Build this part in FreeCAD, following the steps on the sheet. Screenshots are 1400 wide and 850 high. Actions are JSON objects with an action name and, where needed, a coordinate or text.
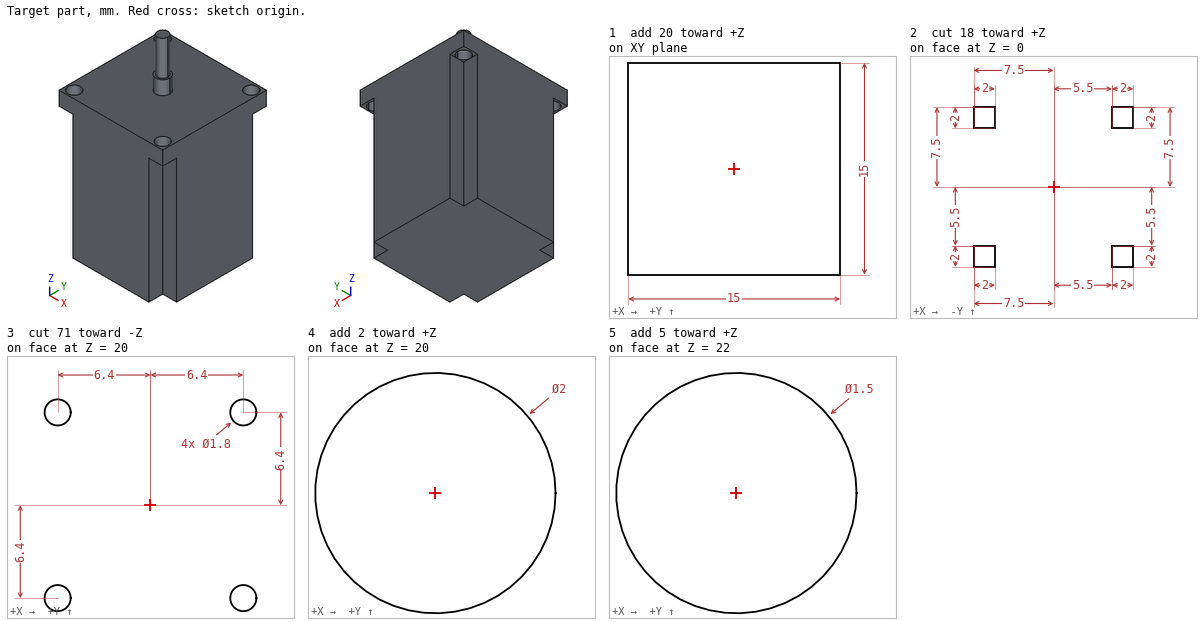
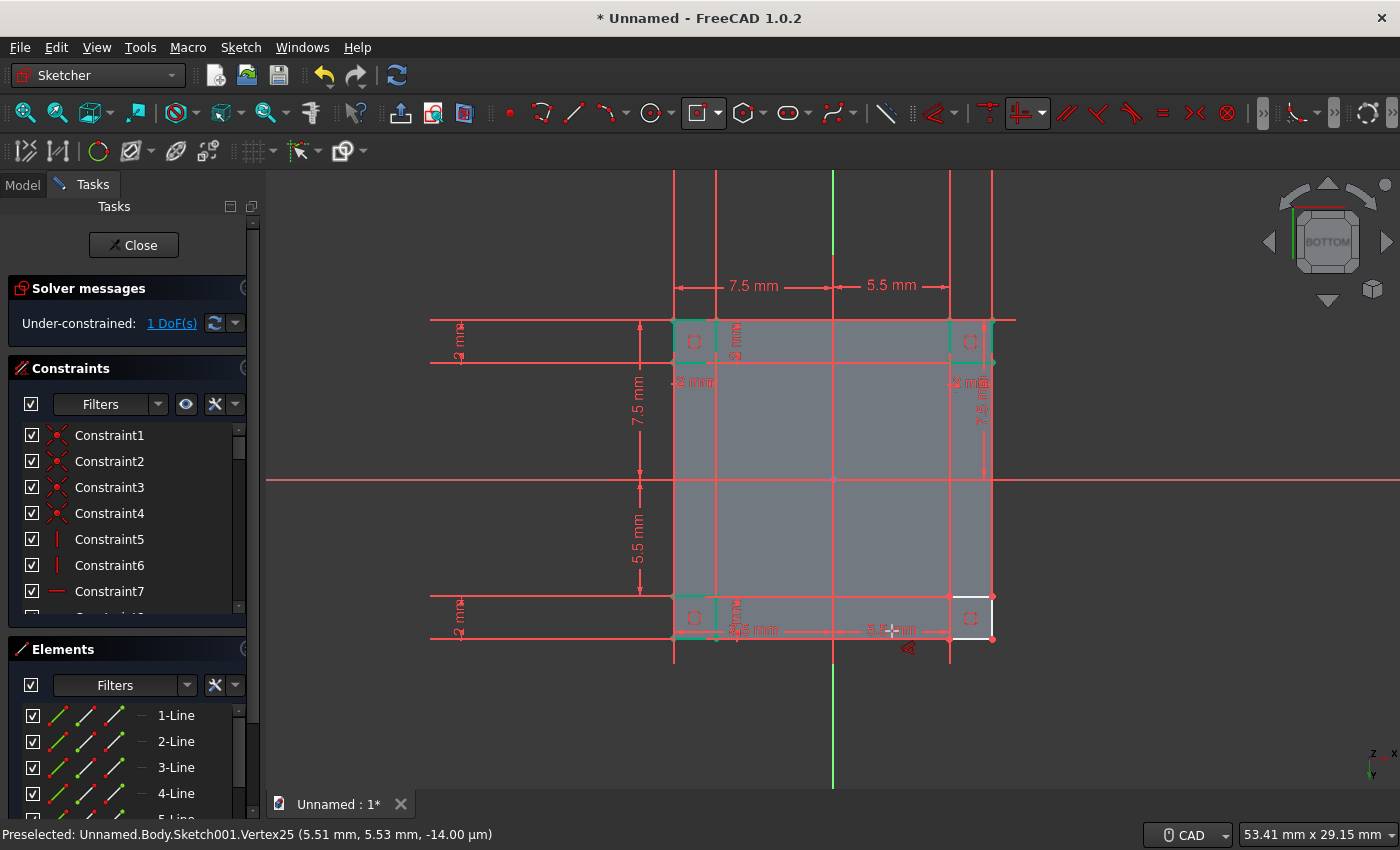
{"action": "left_click", "coordinate": [950, 597]}
{"action": "left_click", "coordinate": [984, 538]}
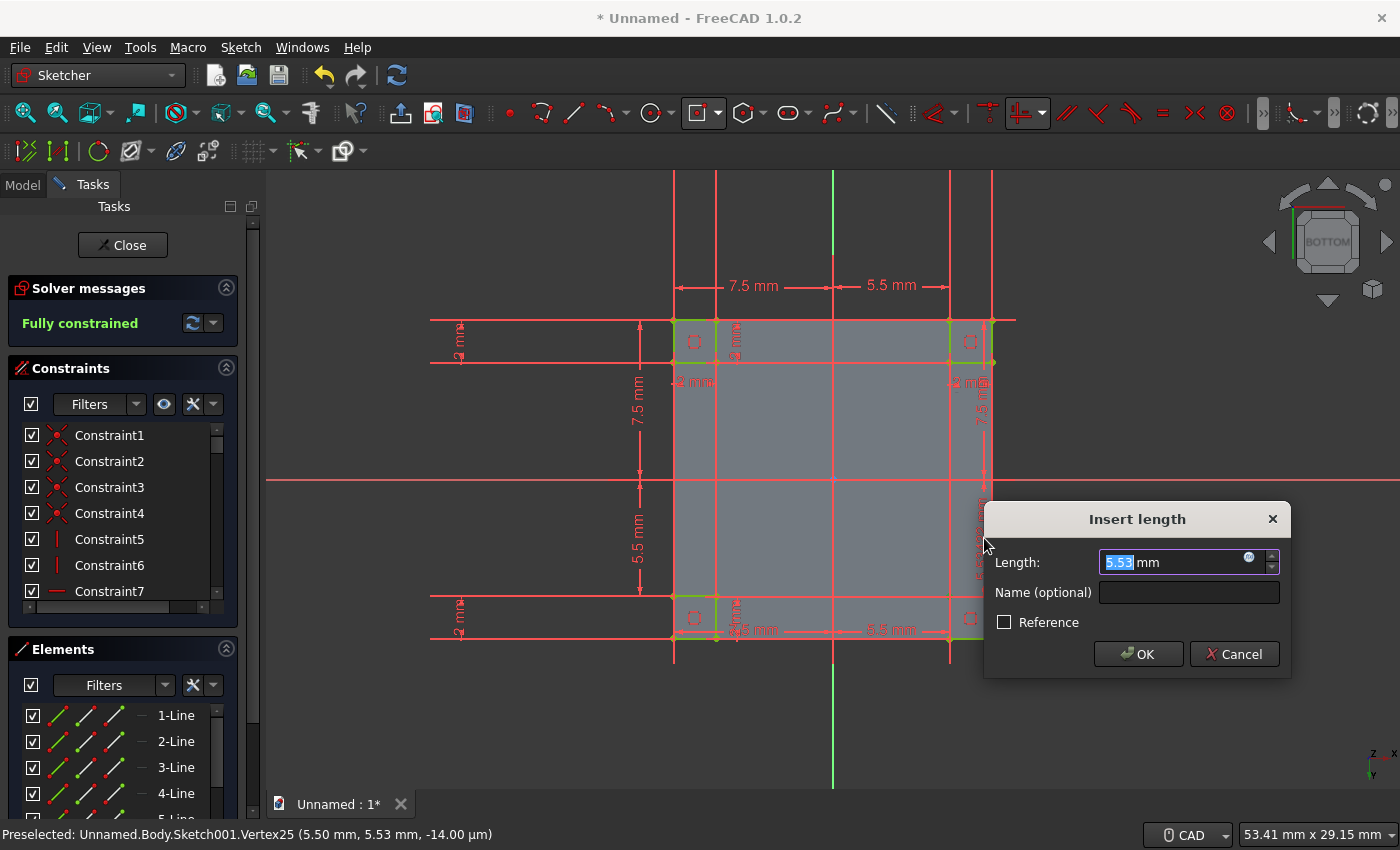
{"action": "type", "text": "5.5"}
{"action": "key", "text": "Return"}
{"action": "key", "text": "Escape"}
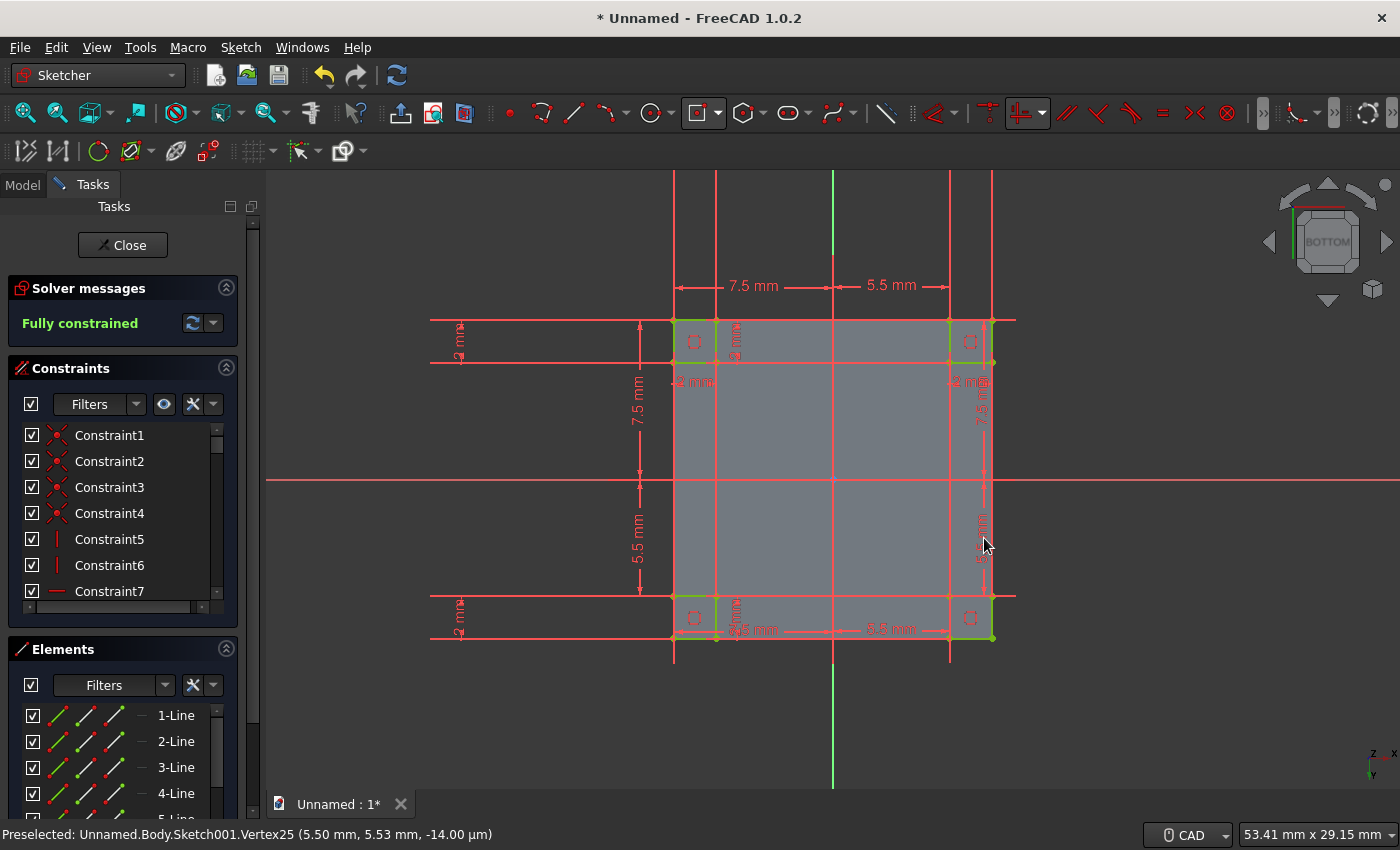
{"action": "left_click", "coordinate": [123, 245]}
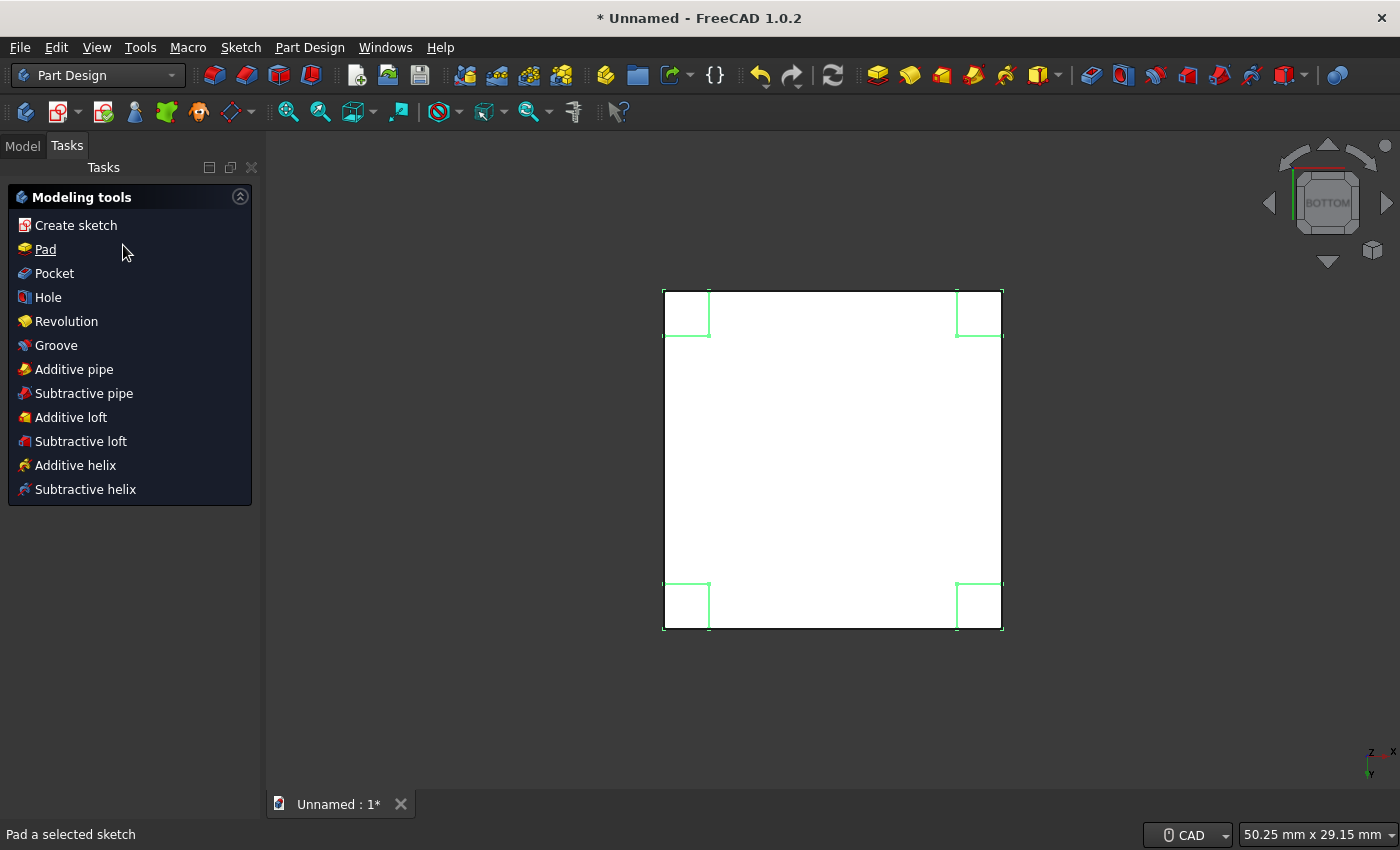
{"action": "left_click", "coordinate": [1092, 76]}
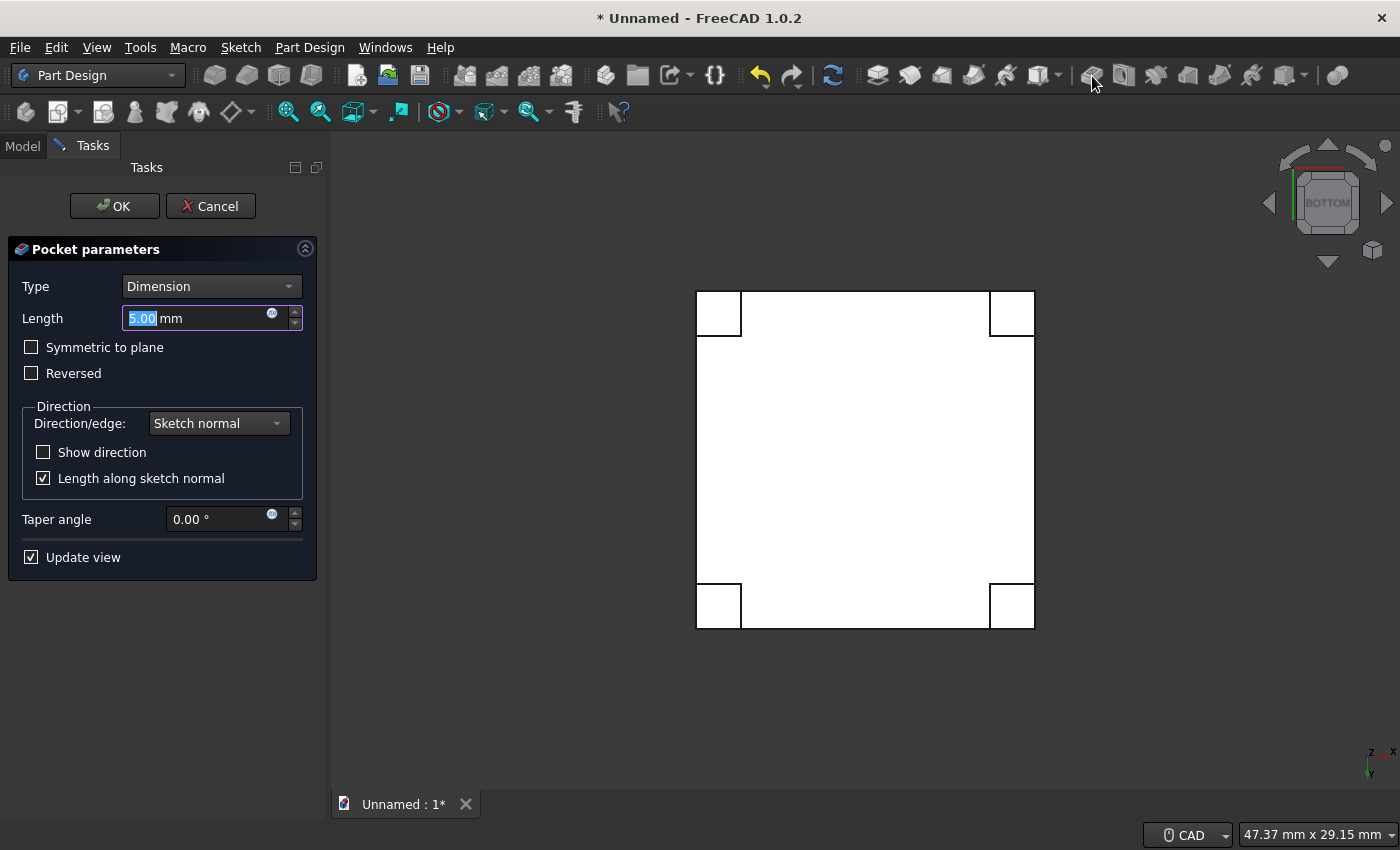
{"action": "type", "text": "18"}
{"action": "key", "text": "Tab"}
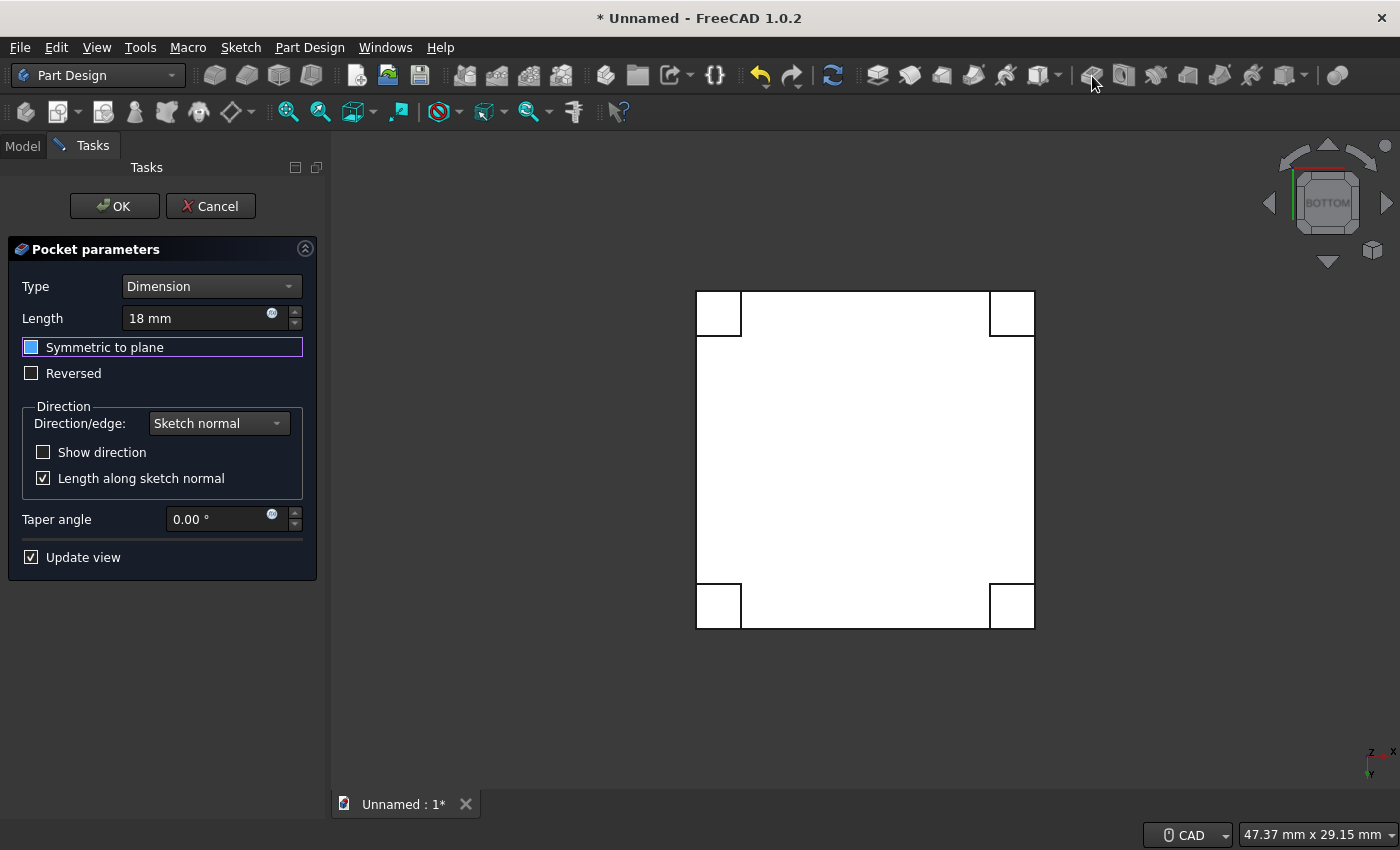
{"action": "left_click", "coordinate": [115, 206]}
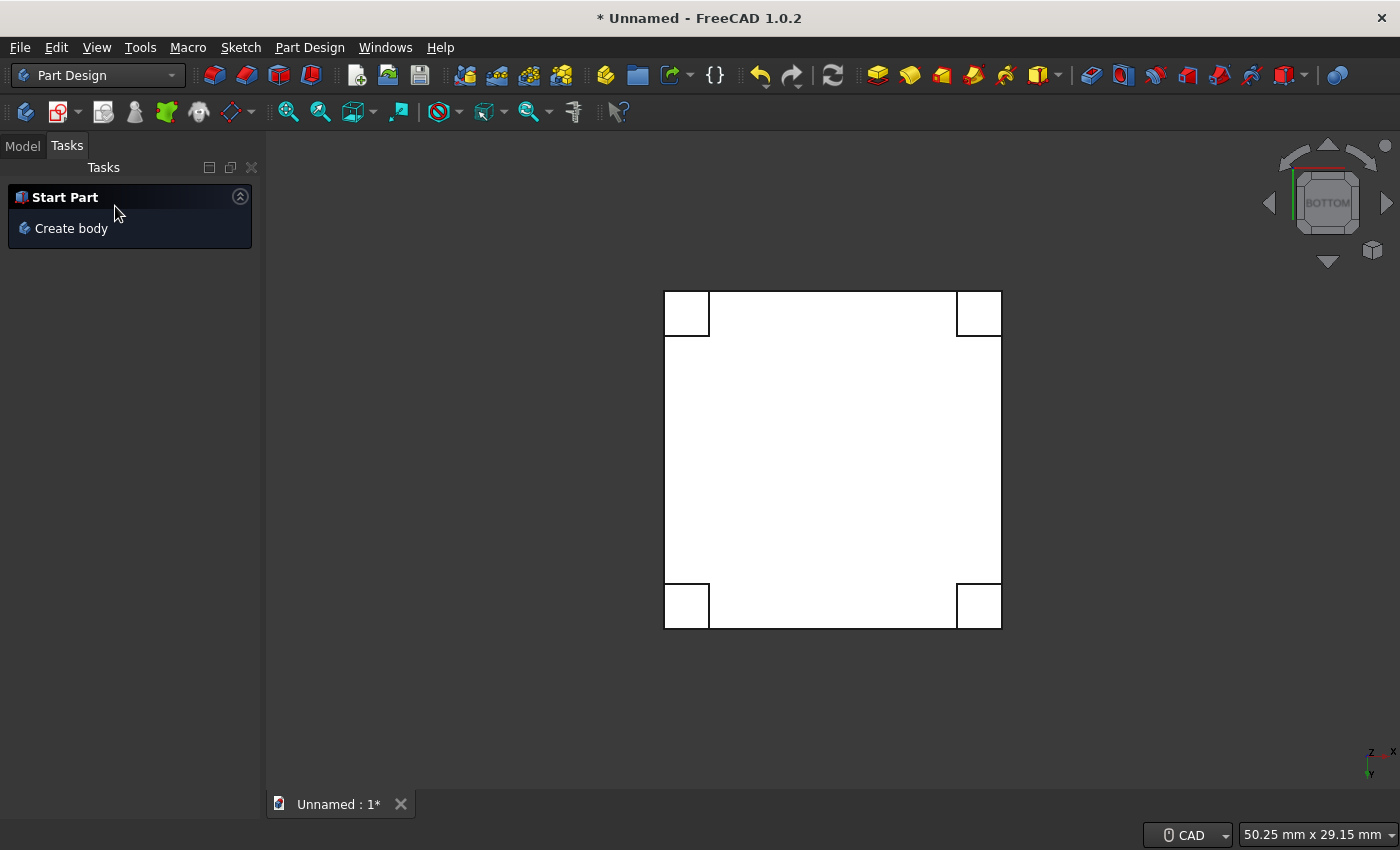
{"action": "key", "text": "0"}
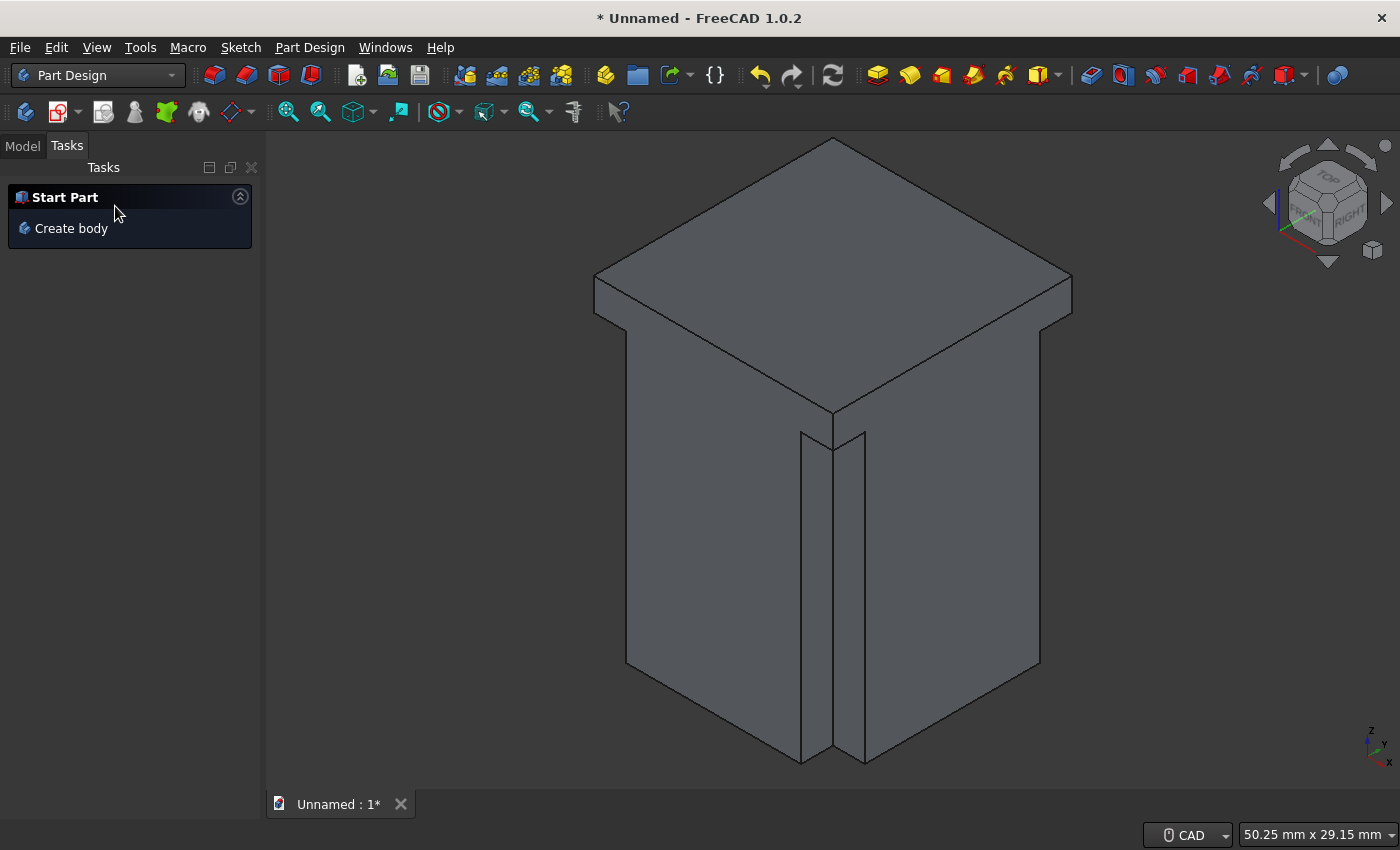
{"action": "left_click", "coordinate": [833, 275]}